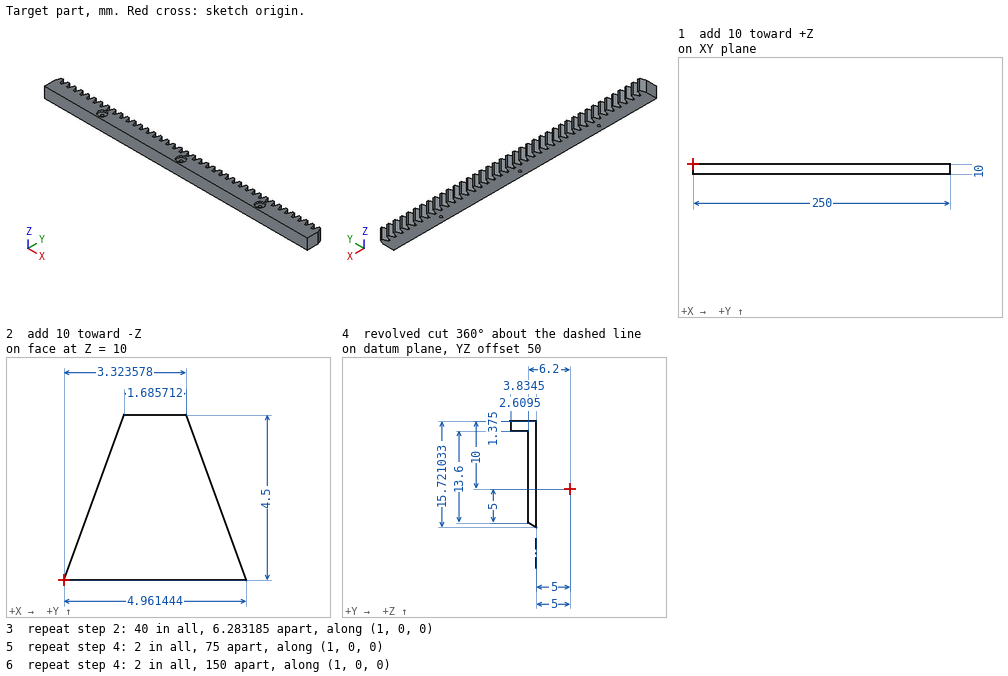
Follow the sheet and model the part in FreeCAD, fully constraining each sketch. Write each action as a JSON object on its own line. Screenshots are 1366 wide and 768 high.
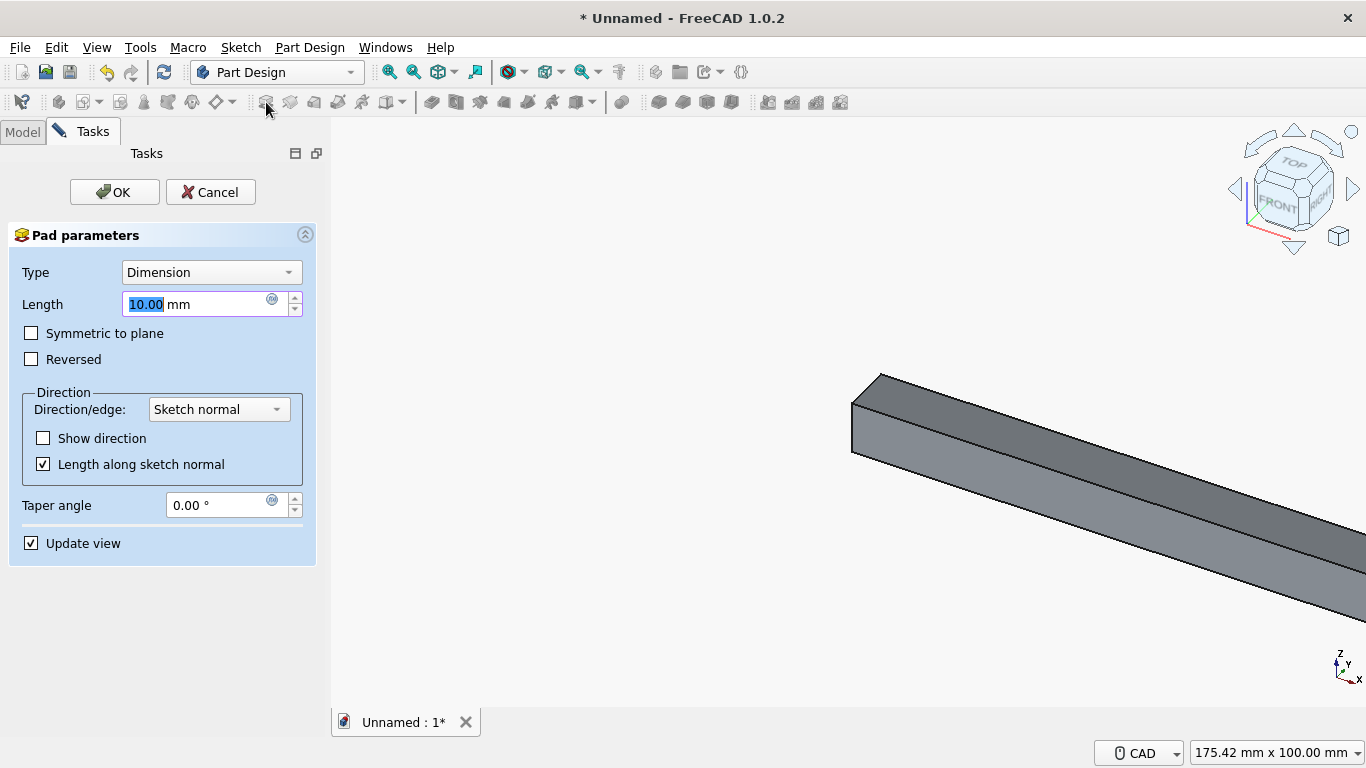
{"action": "type", "text": "10"}
{"action": "key", "text": "Tab"}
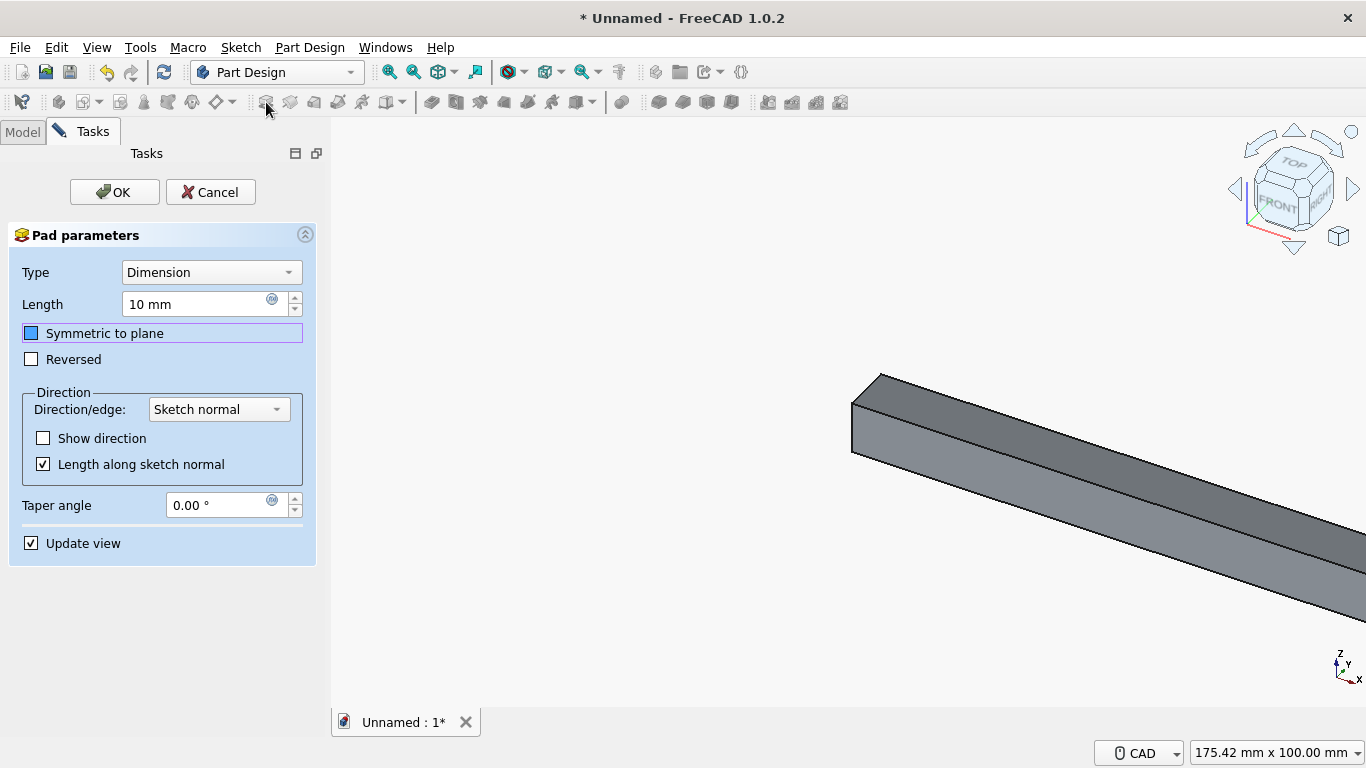
{"action": "left_click", "coordinate": [115, 192]}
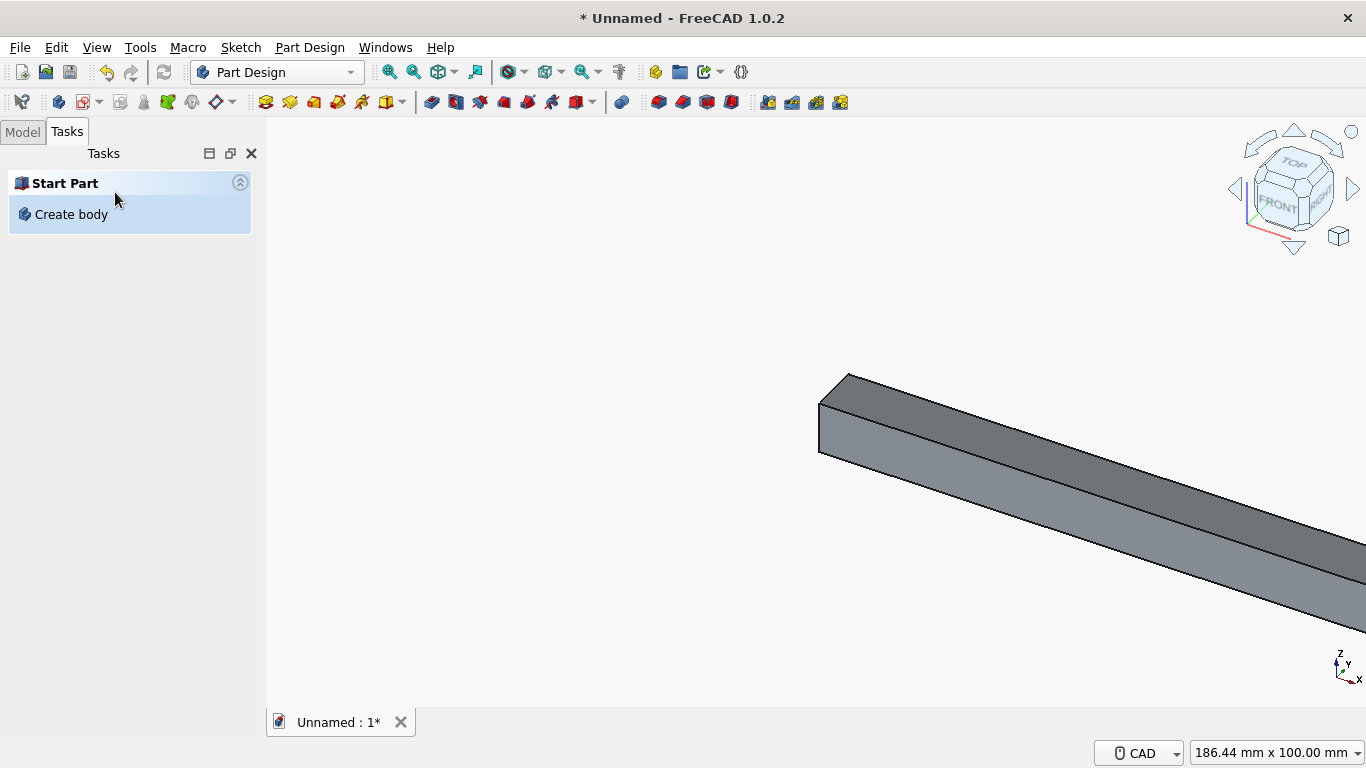
{"action": "key", "text": "v f"}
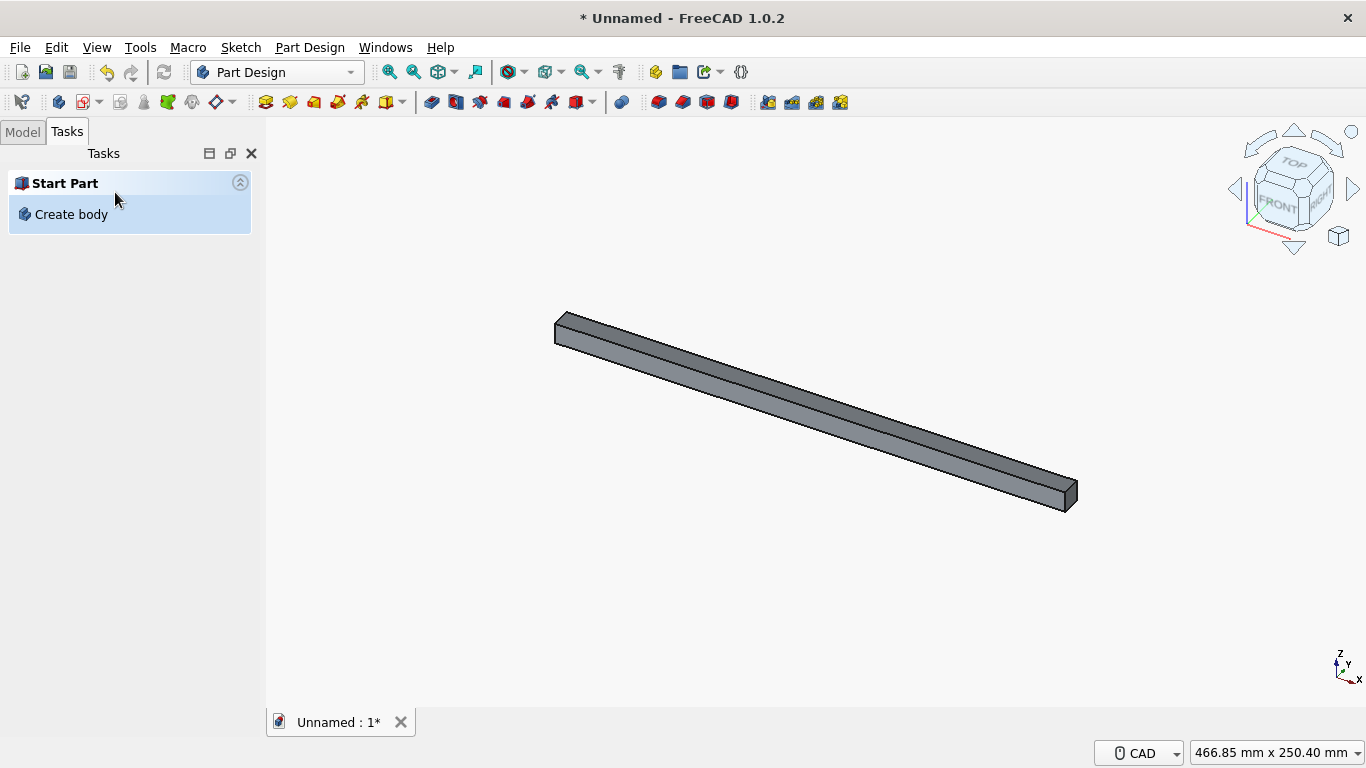
{"action": "left_click", "coordinate": [1036, 472]}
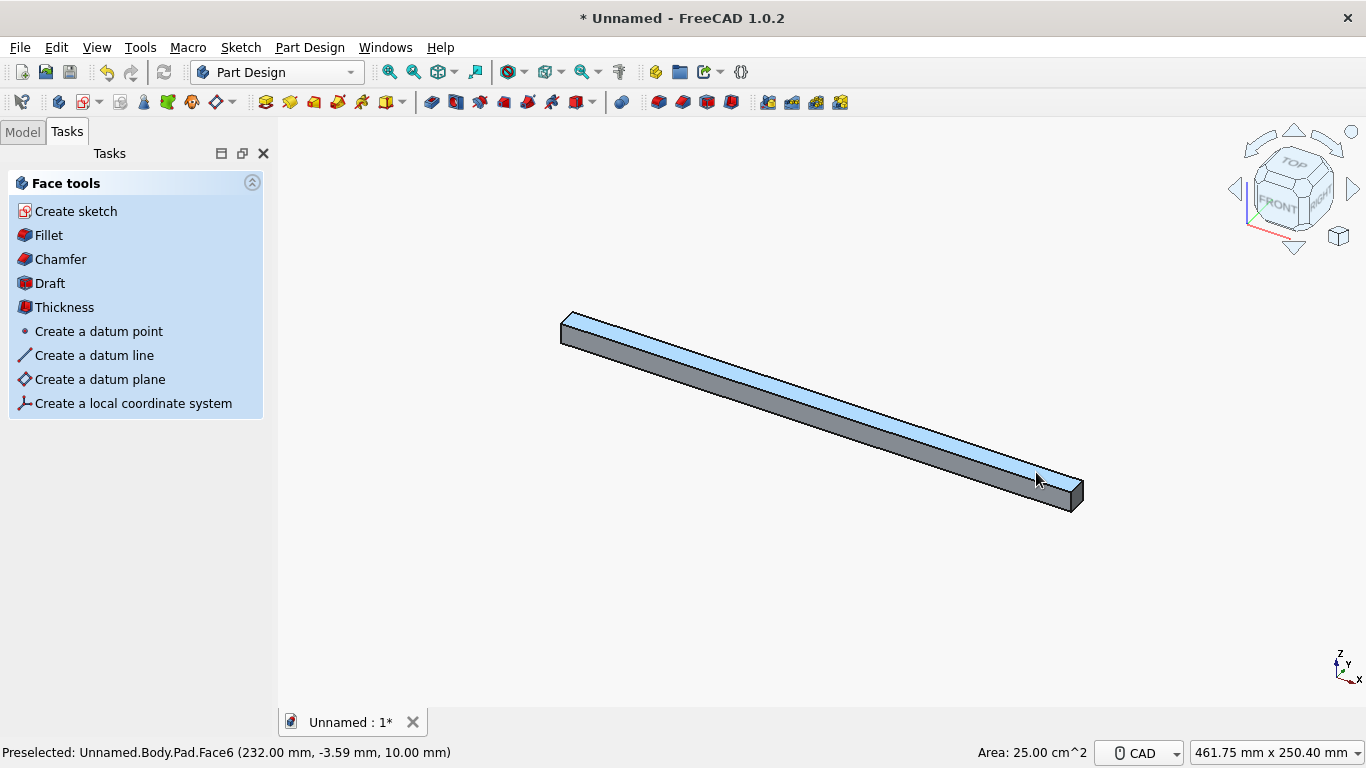
{"action": "left_click", "coordinate": [84, 102]}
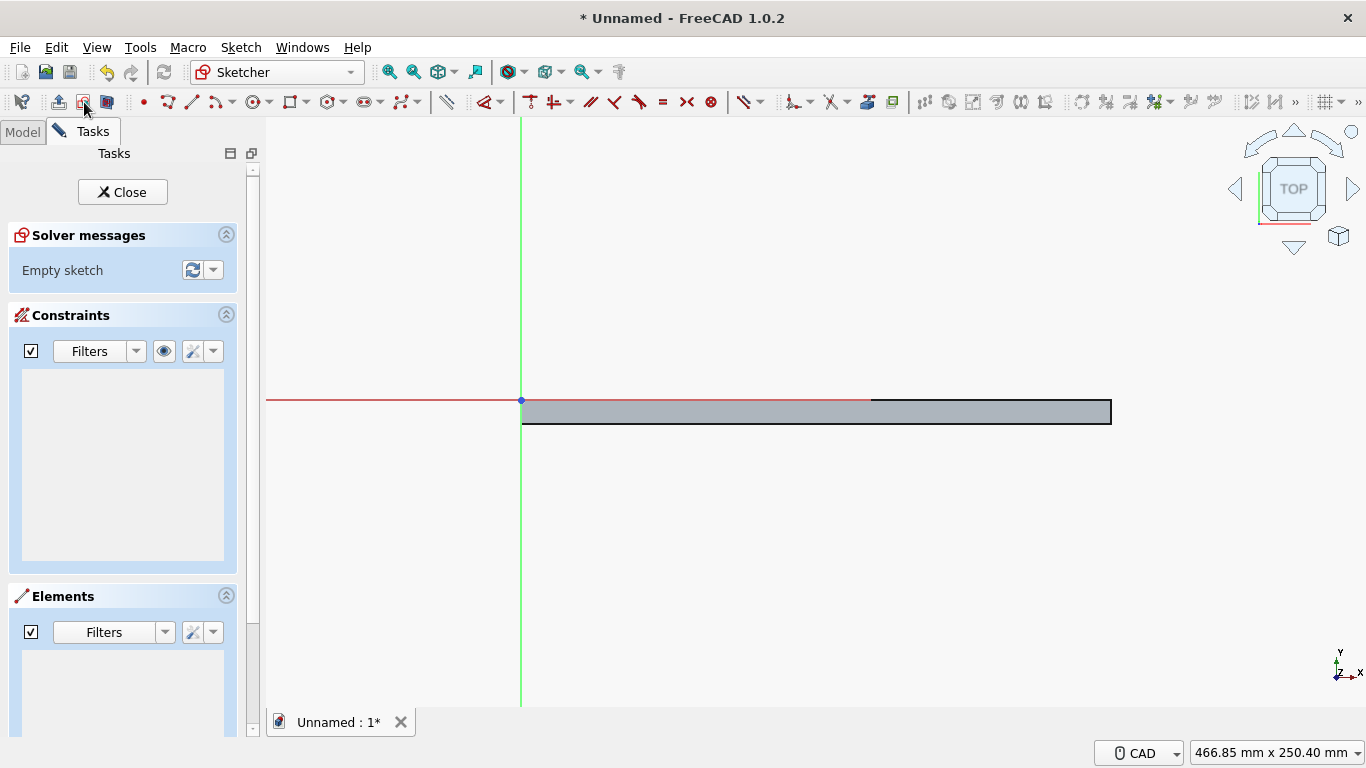
{"action": "scroll", "coordinate": [516, 394], "scroll_direction": "up", "scroll_amount": 15}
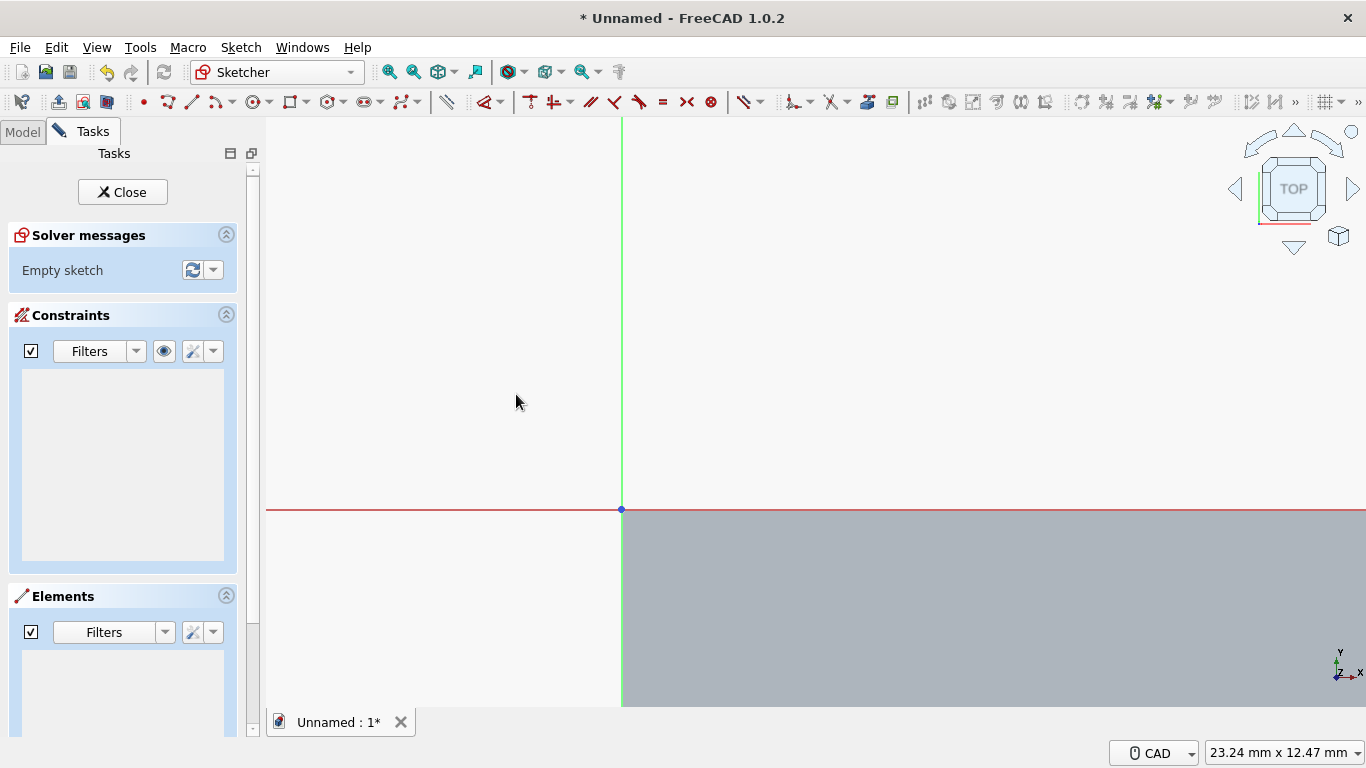
{"action": "scroll", "coordinate": [729, 393], "scroll_direction": "up", "scroll_amount": 3}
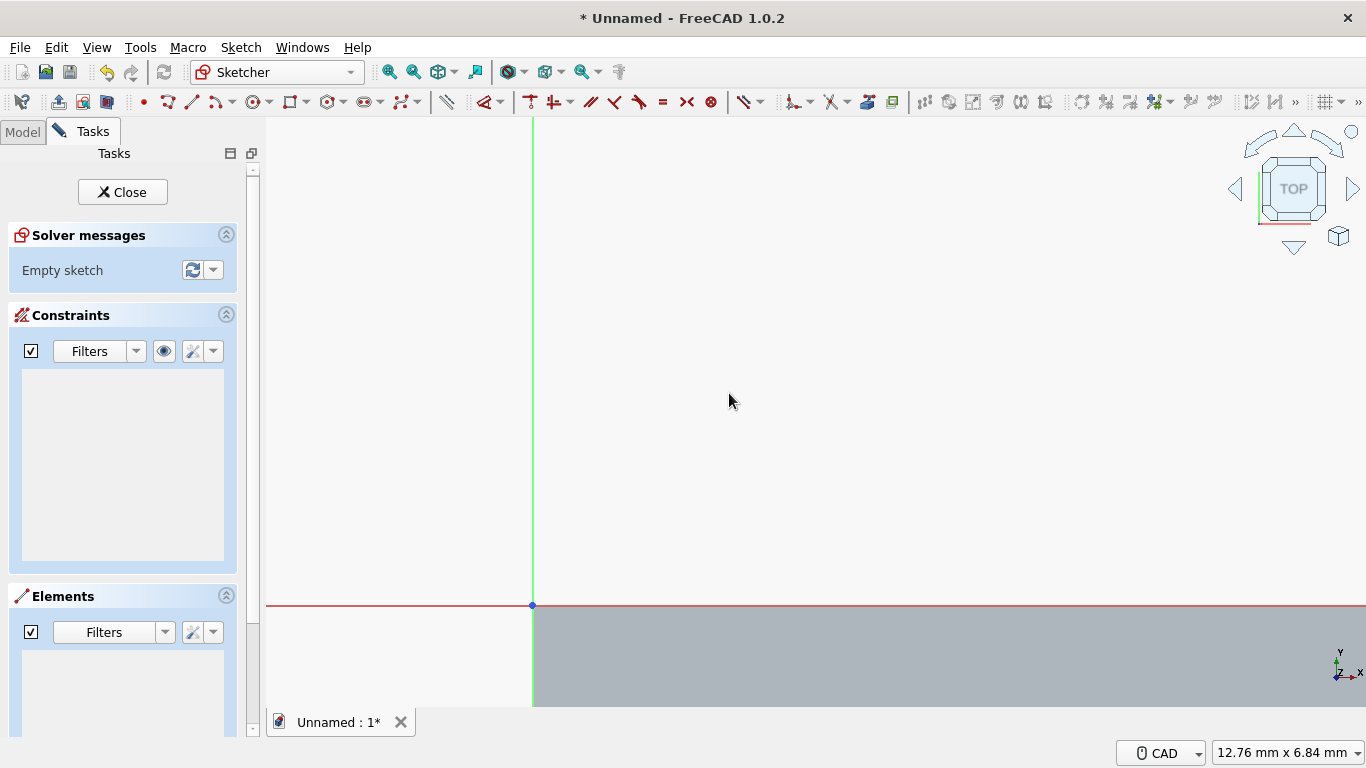
{"action": "left_click", "coordinate": [168, 102]}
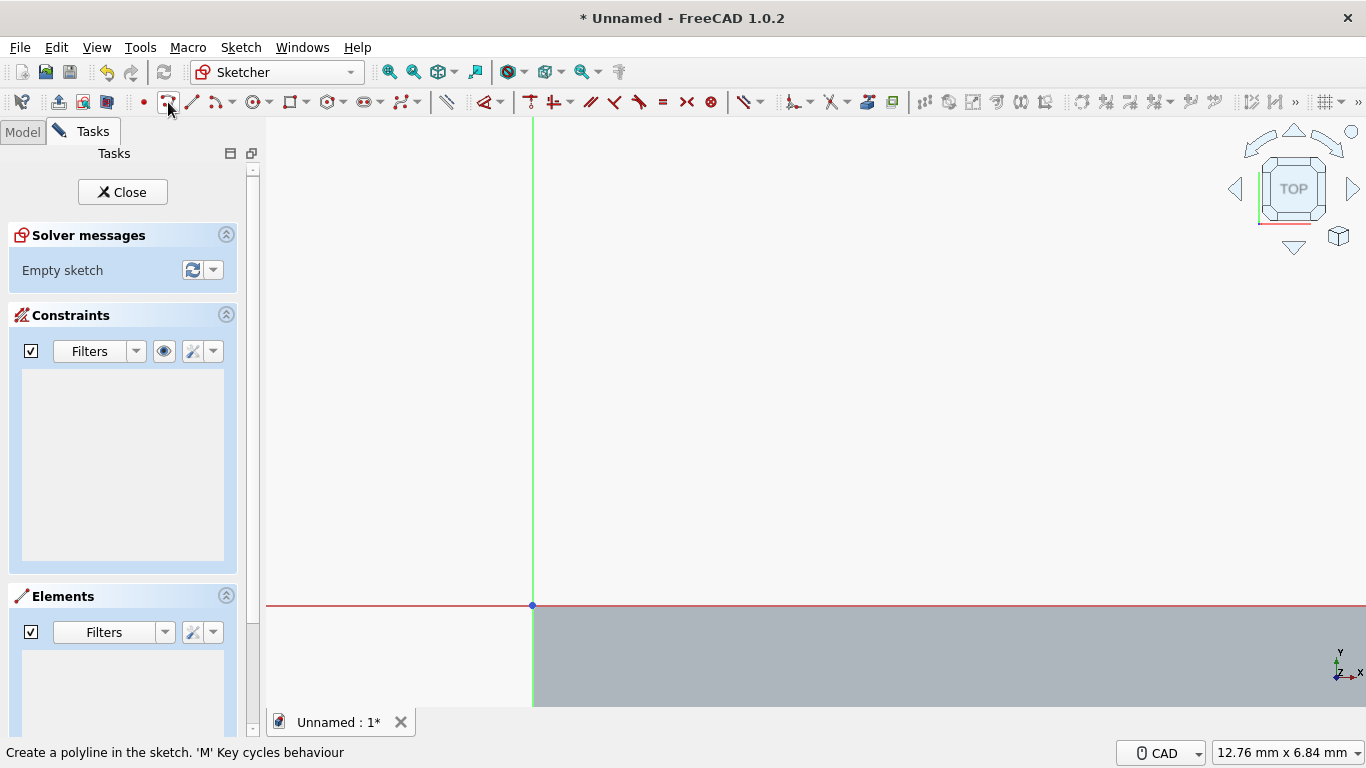
{"action": "left_click", "coordinate": [533, 606]}
{"action": "left_click", "coordinate": [961, 597]}
{"action": "left_click", "coordinate": [819, 218]}
{"action": "left_click", "coordinate": [674, 218]}
{"action": "left_click", "coordinate": [533, 606]}
{"action": "key", "text": "Escape"}
{"action": "key", "text": "Escape"}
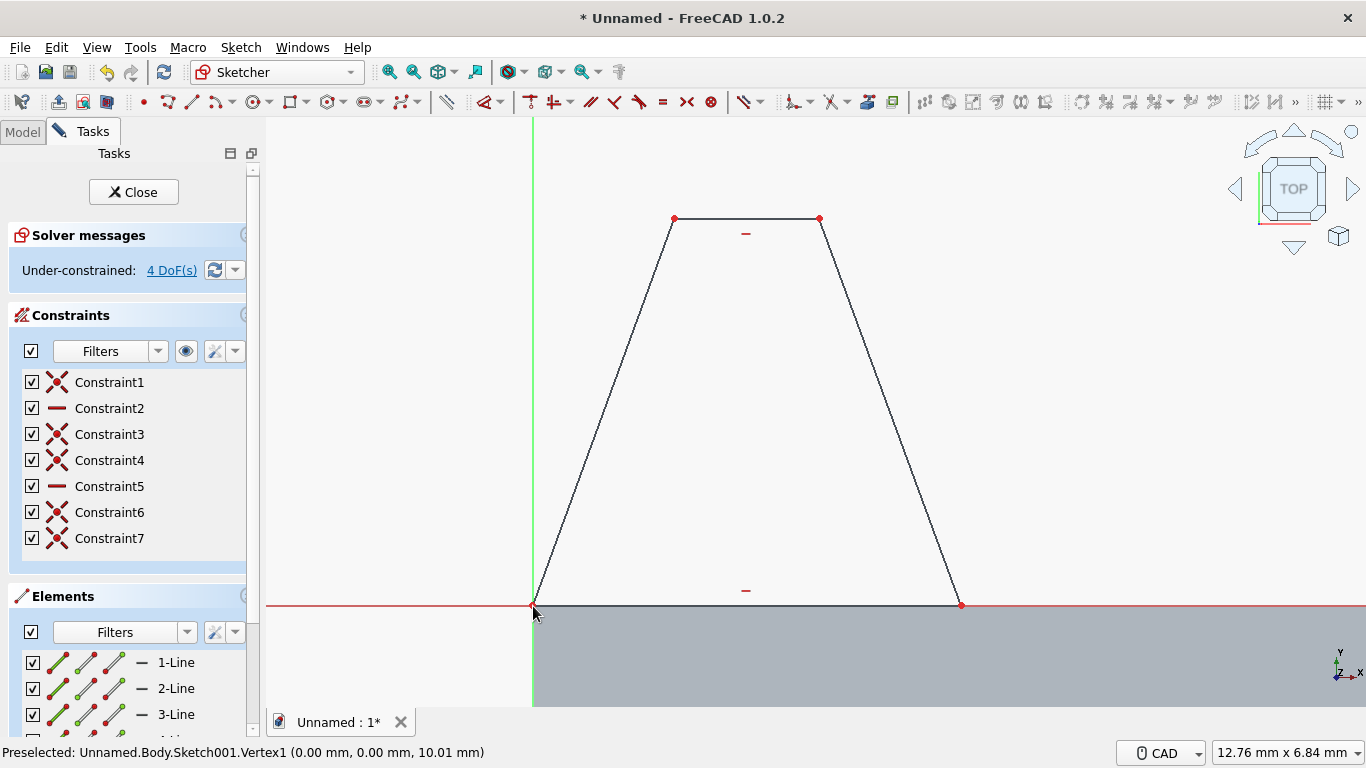
{"action": "key", "text": "d"}